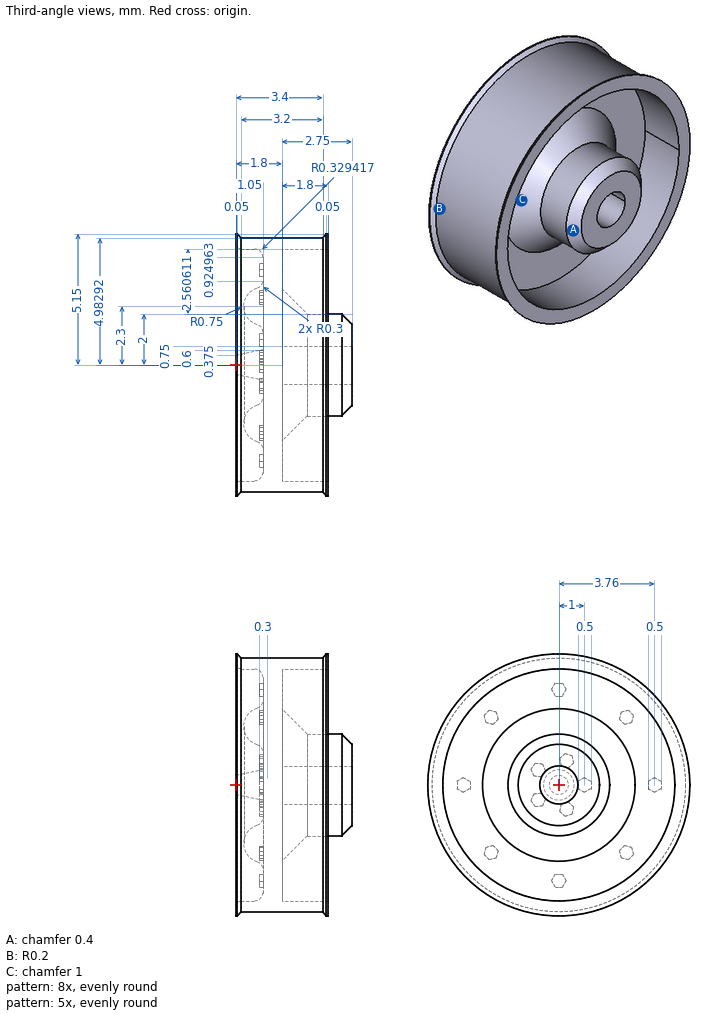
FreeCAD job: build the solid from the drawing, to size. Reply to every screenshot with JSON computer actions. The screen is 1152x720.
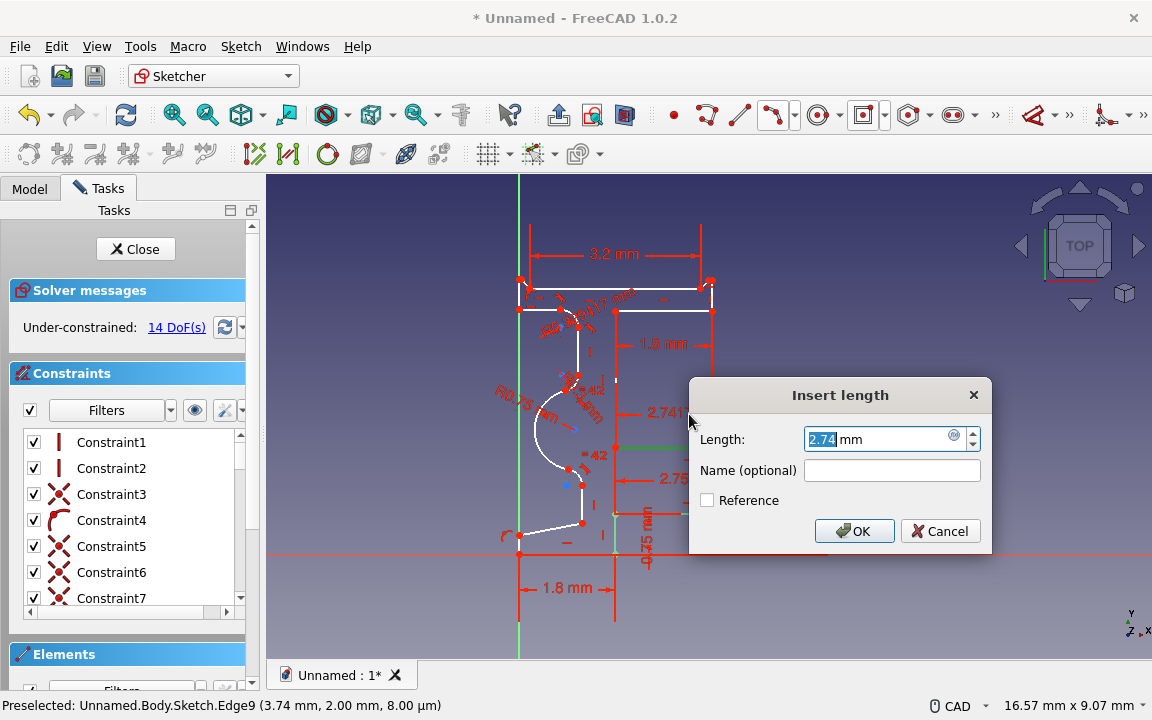
{"action": "type", "text": "2.75"}
{"action": "key", "text": "Return"}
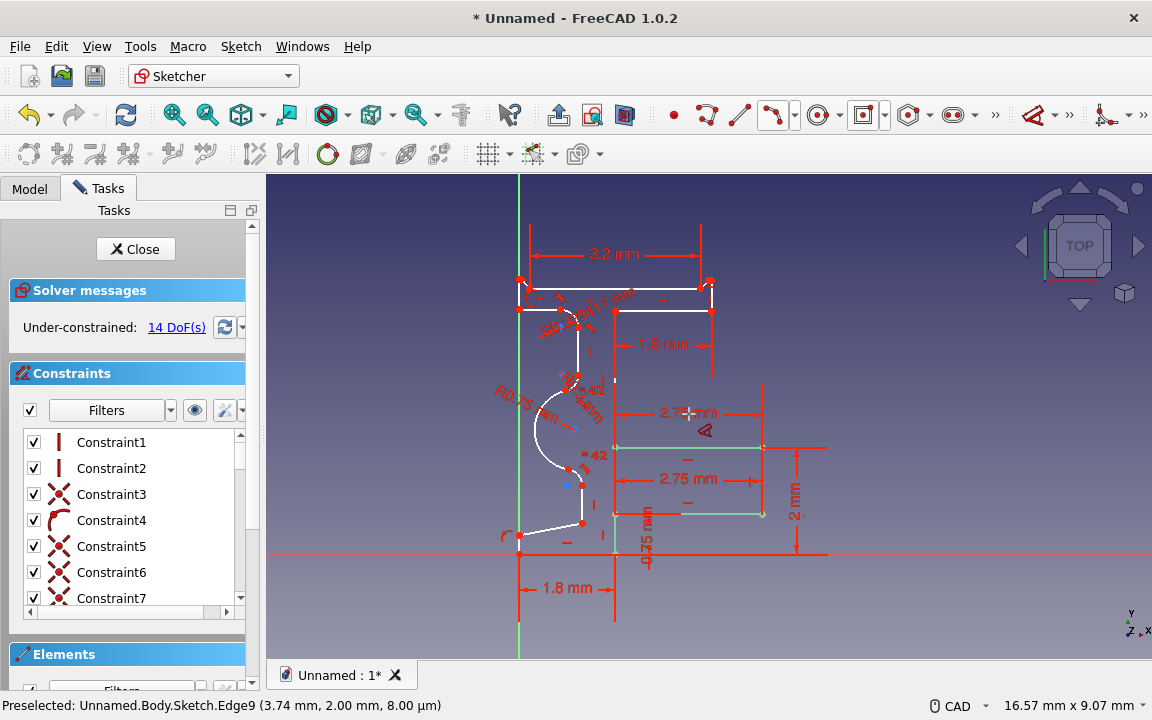
{"action": "scroll", "coordinate": [710, 280], "scroll_direction": "up", "scroll_amount": 14}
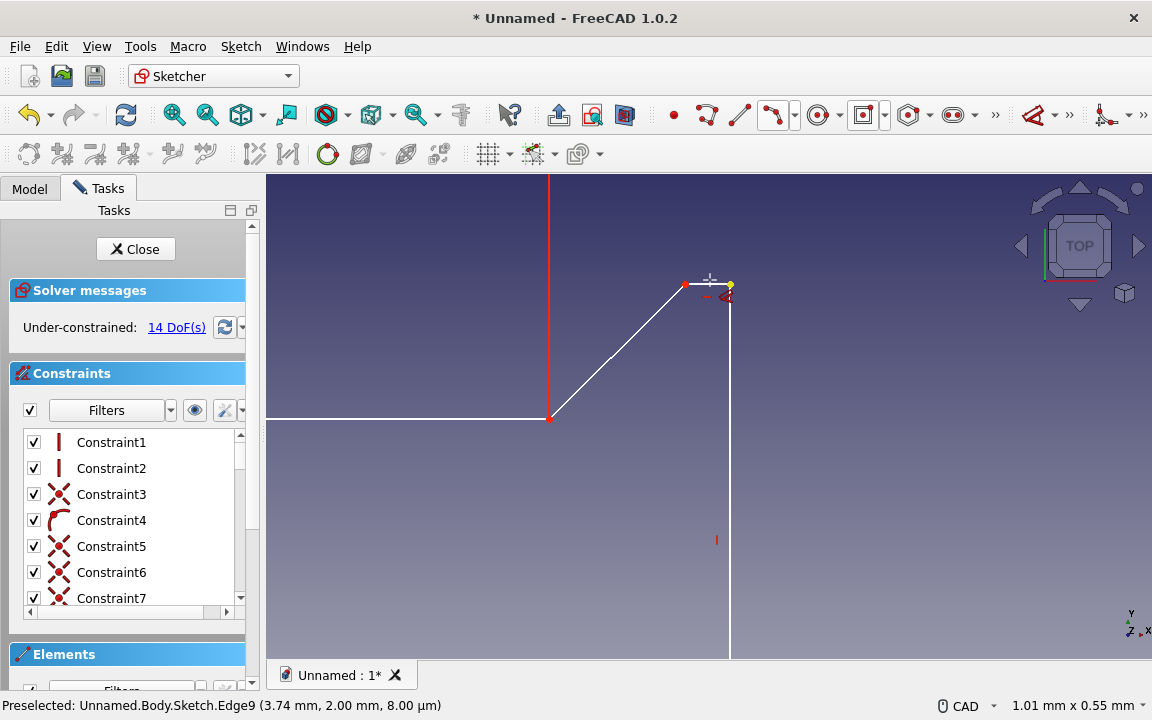
{"action": "left_click", "coordinate": [708, 284]}
{"action": "left_click", "coordinate": [708, 250]}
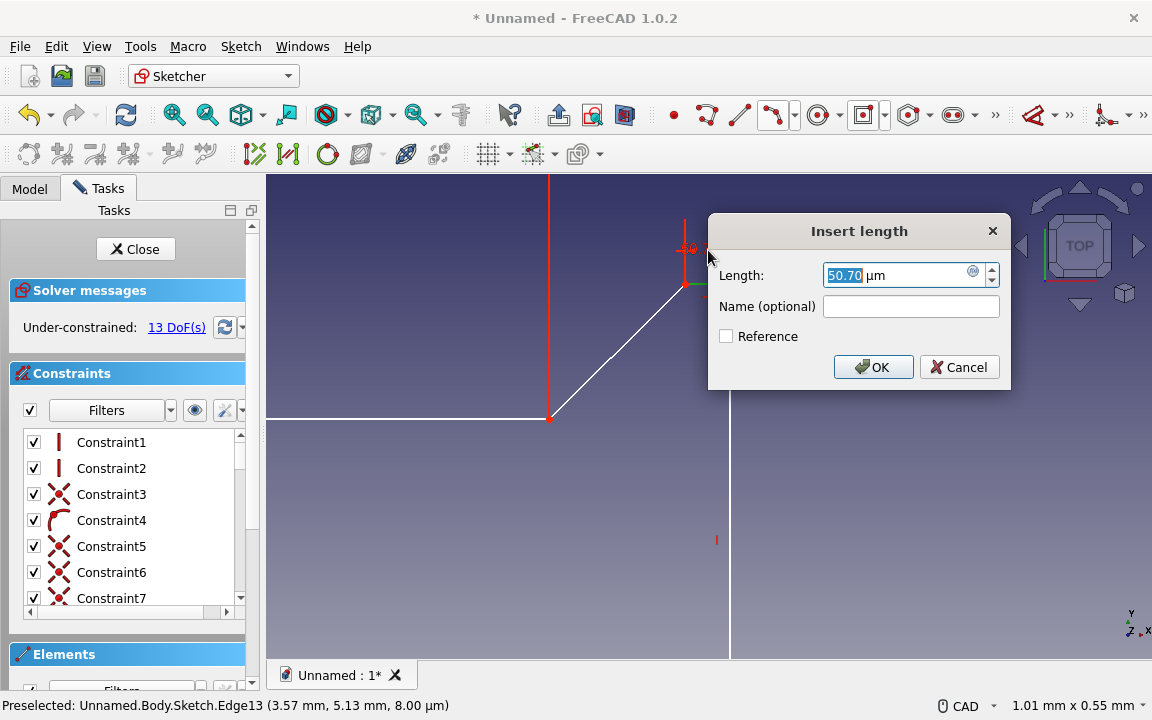
{"action": "key", "text": "ctrl+a"}
{"action": "type", "text": "0.05 mm"}
{"action": "key", "text": "Return"}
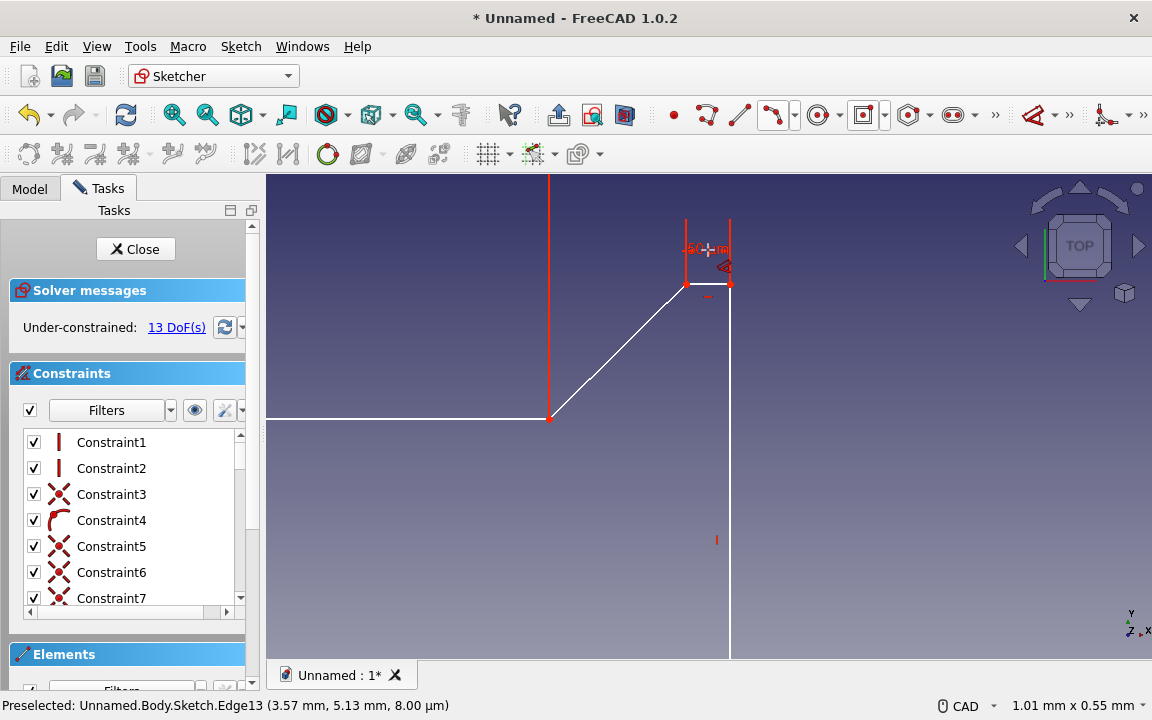
{"action": "scroll", "coordinate": [710, 280], "scroll_direction": "down", "scroll_amount": 14}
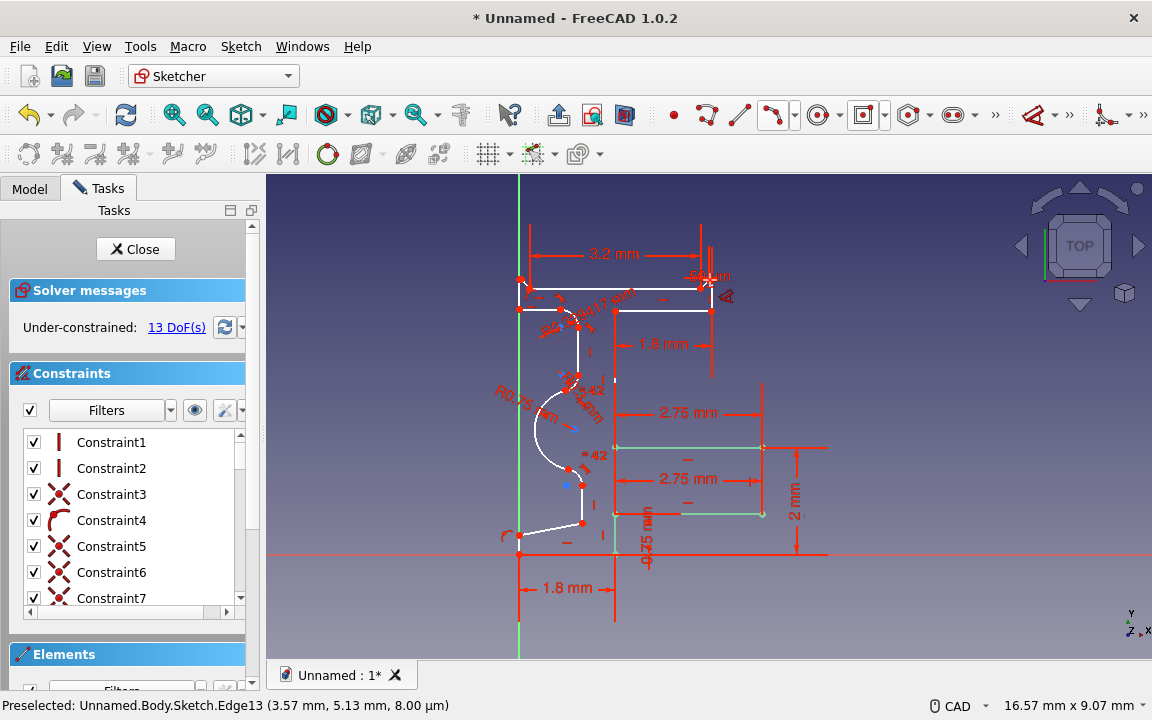
{"action": "scroll", "coordinate": [521, 279], "scroll_direction": "up", "scroll_amount": 14}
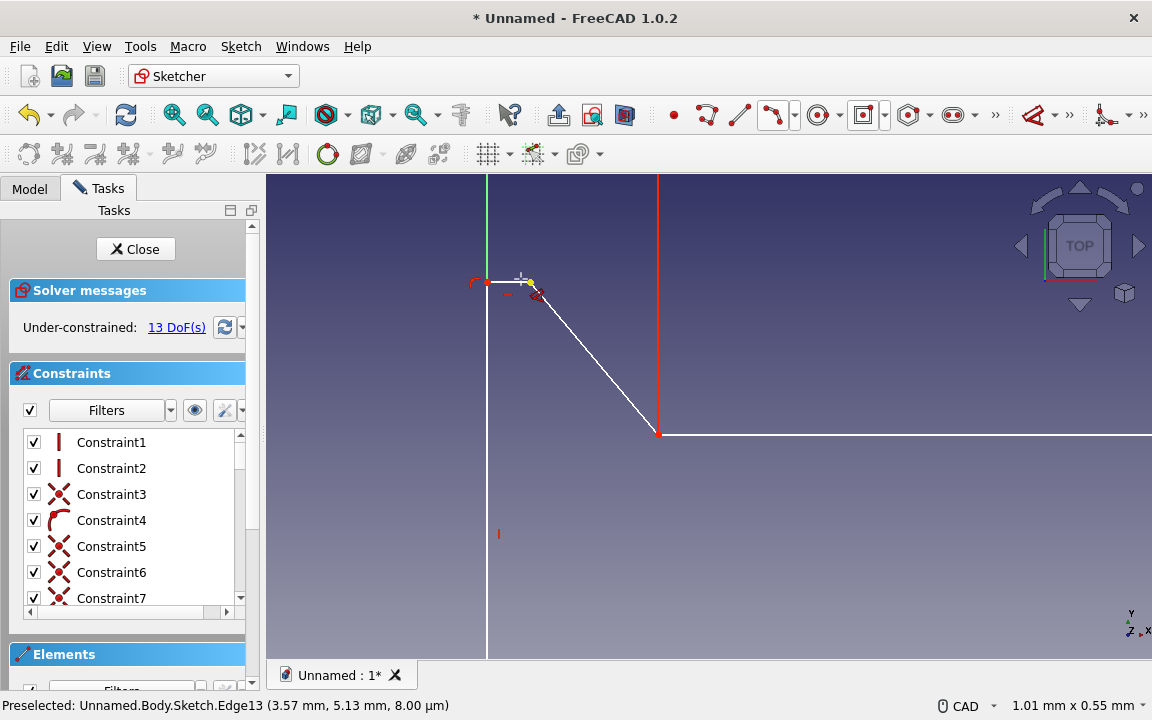
{"action": "left_click", "coordinate": [517, 282]}
{"action": "left_click", "coordinate": [509, 248]}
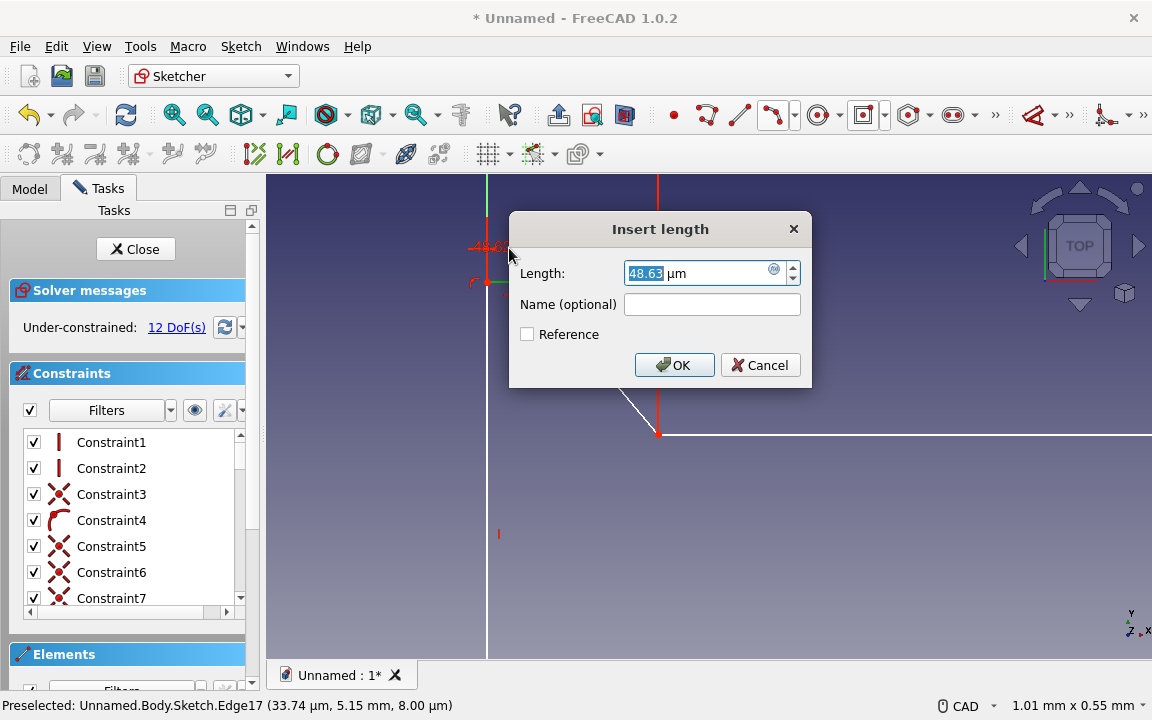
{"action": "key", "text": "ctrl+a"}
{"action": "type", "text": "0.05 mm"}
{"action": "key", "text": "Return"}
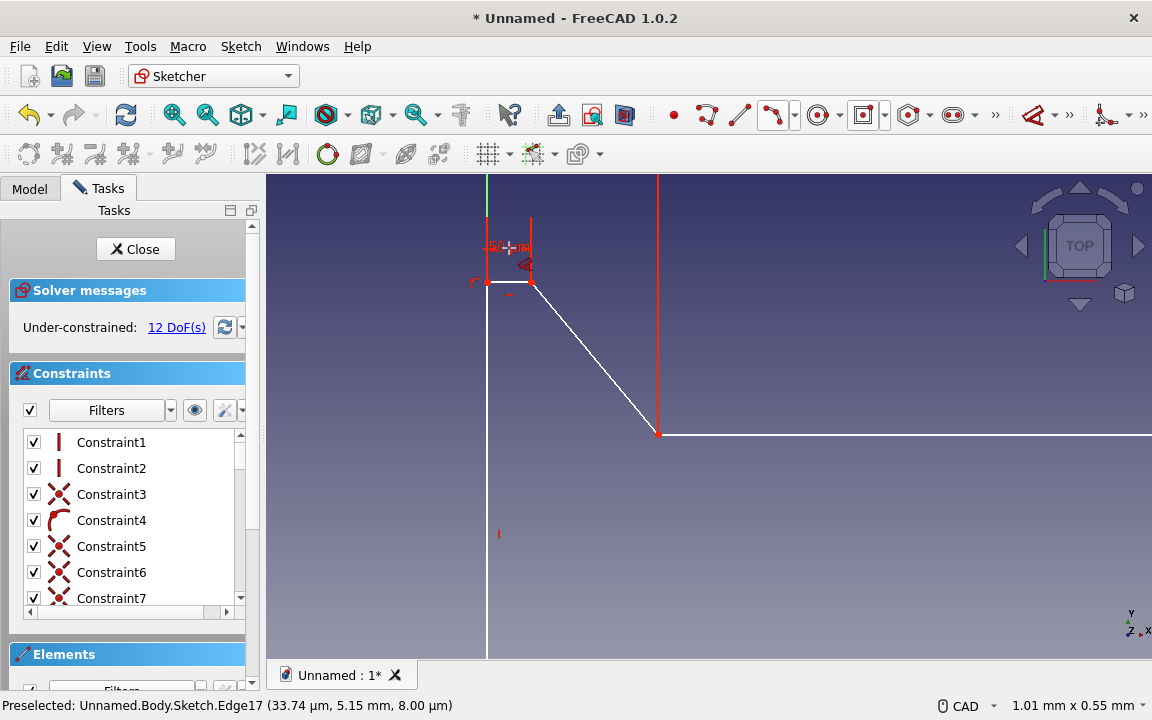
{"action": "scroll", "coordinate": [521, 279], "scroll_direction": "down", "scroll_amount": 14}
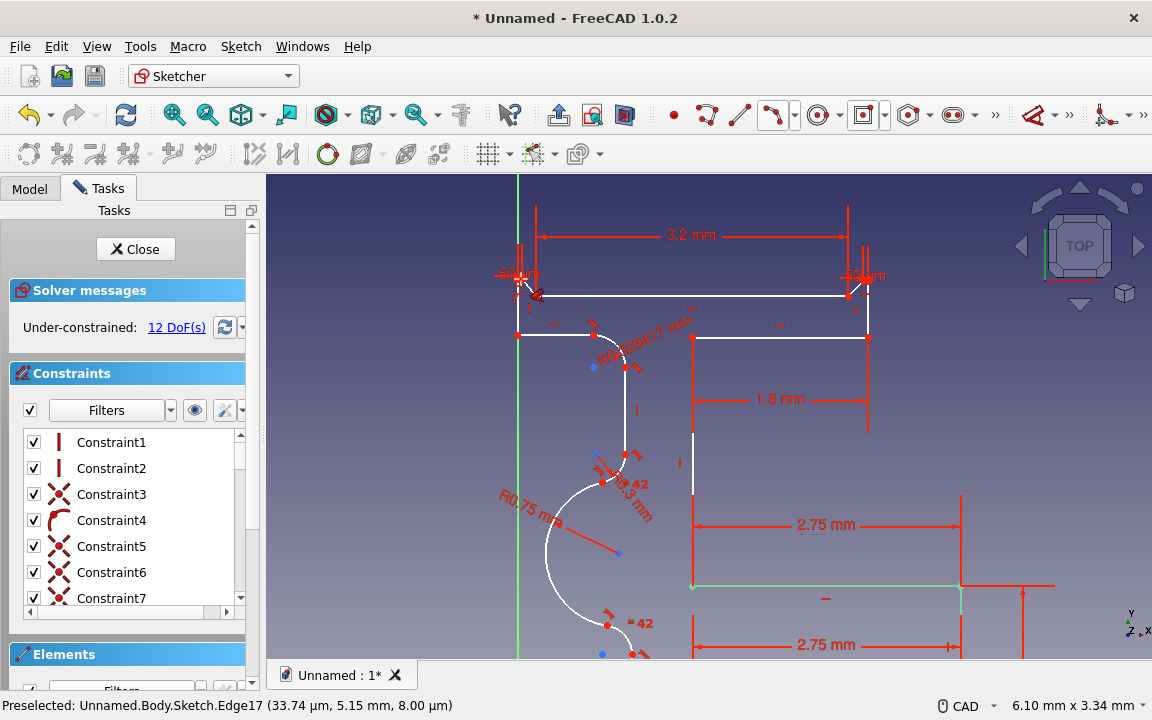
{"action": "scroll", "coordinate": [582, 523], "scroll_direction": "up", "scroll_amount": 2}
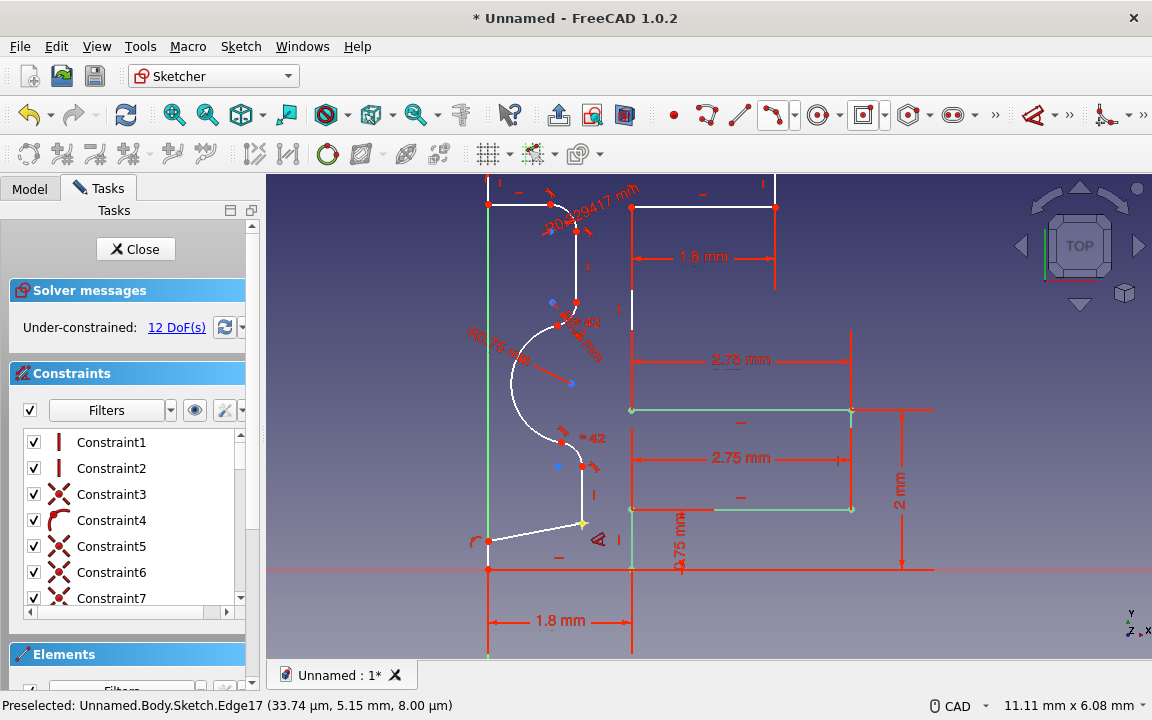
{"action": "left_click", "coordinate": [582, 523]}
{"action": "left_click", "coordinate": [454, 547]}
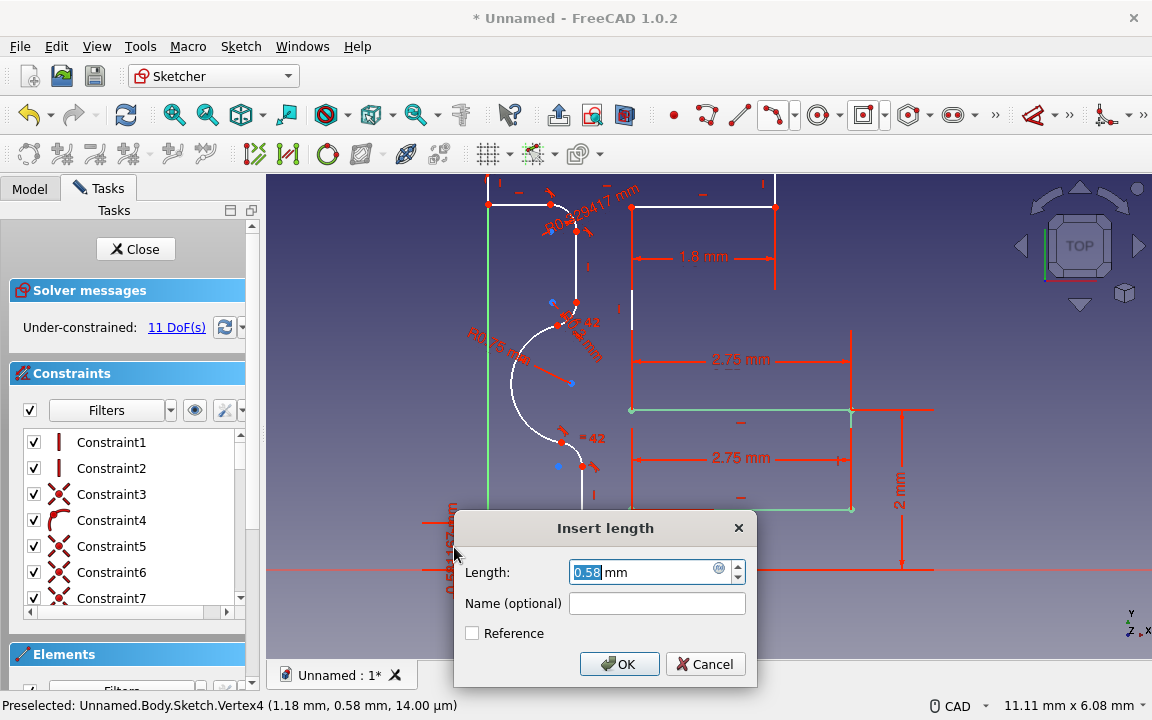
{"action": "type", "text": "0.6"}
{"action": "key", "text": "Return"}